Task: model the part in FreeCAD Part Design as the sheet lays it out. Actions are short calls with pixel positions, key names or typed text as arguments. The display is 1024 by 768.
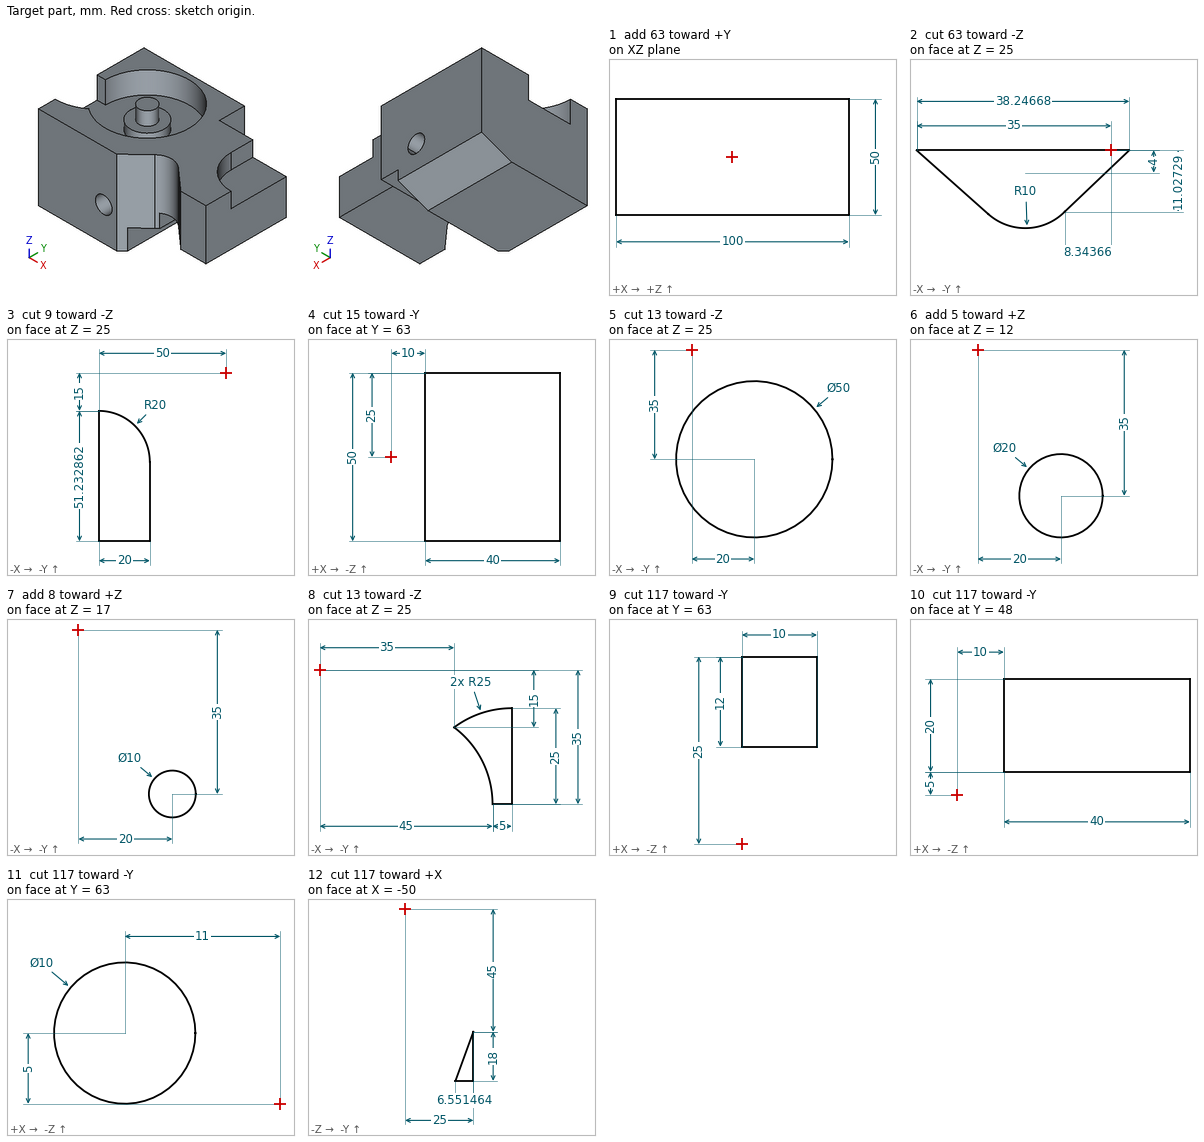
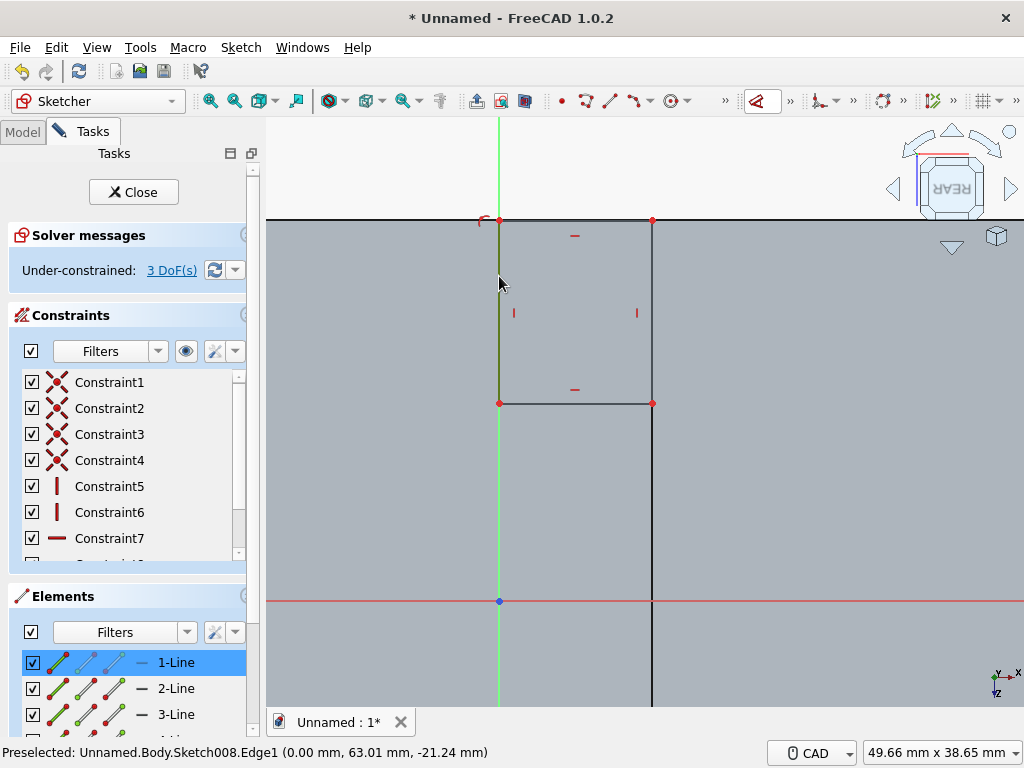
click(776, 102)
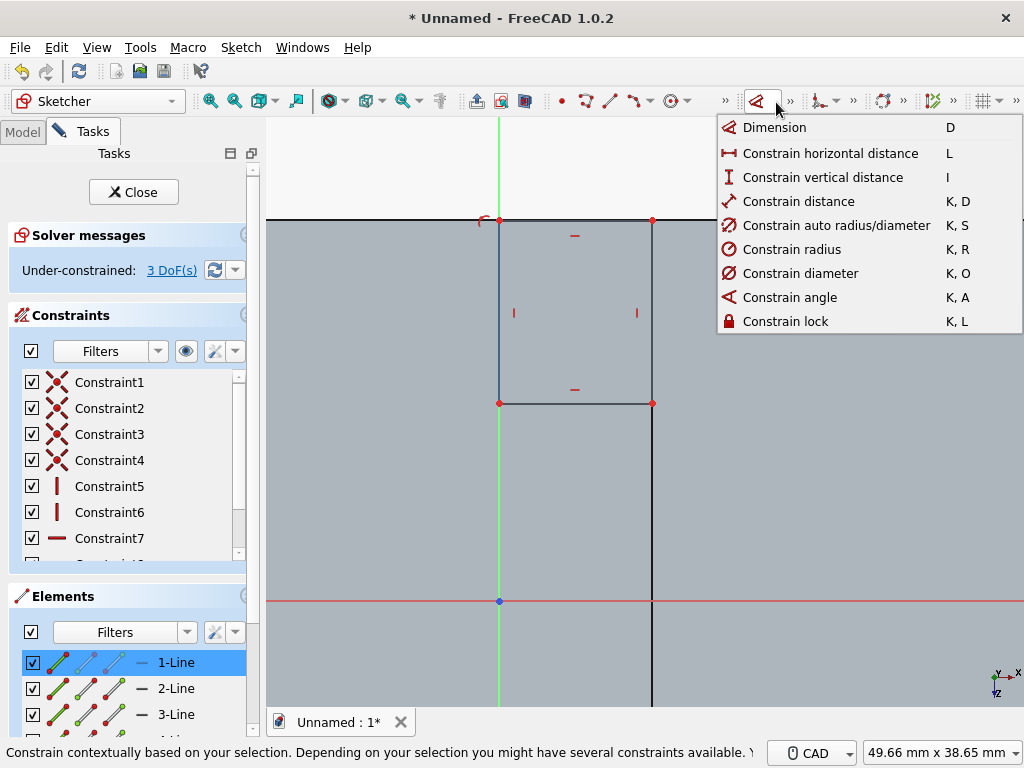
click(870, 177)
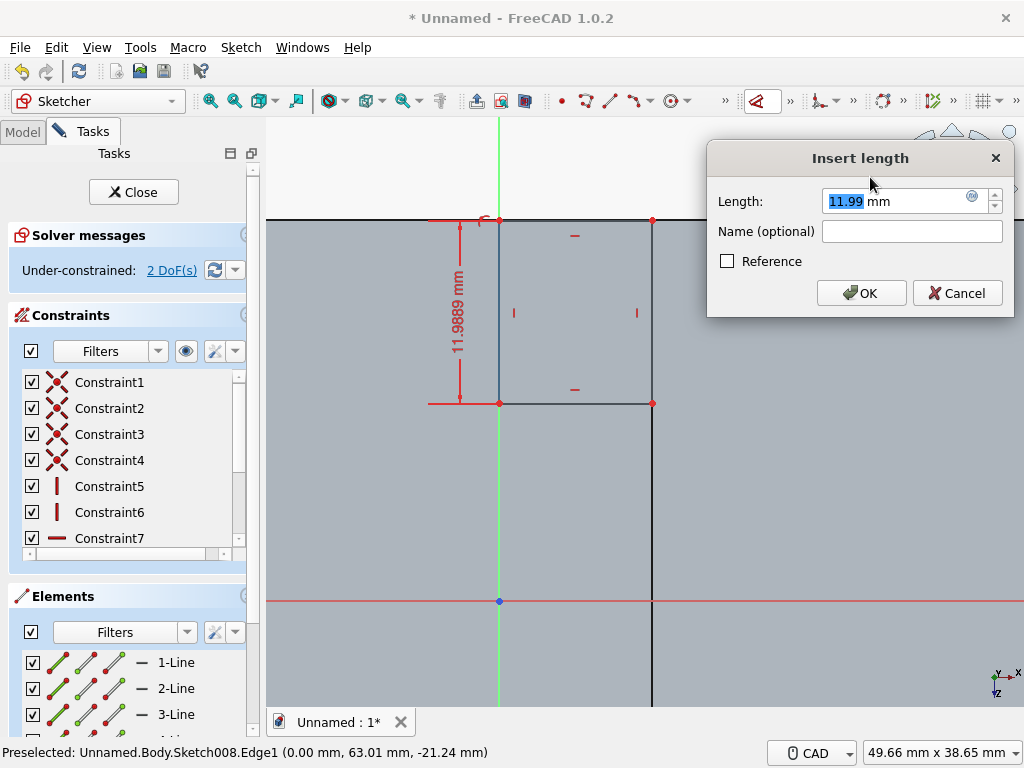
text(12)
key(Return)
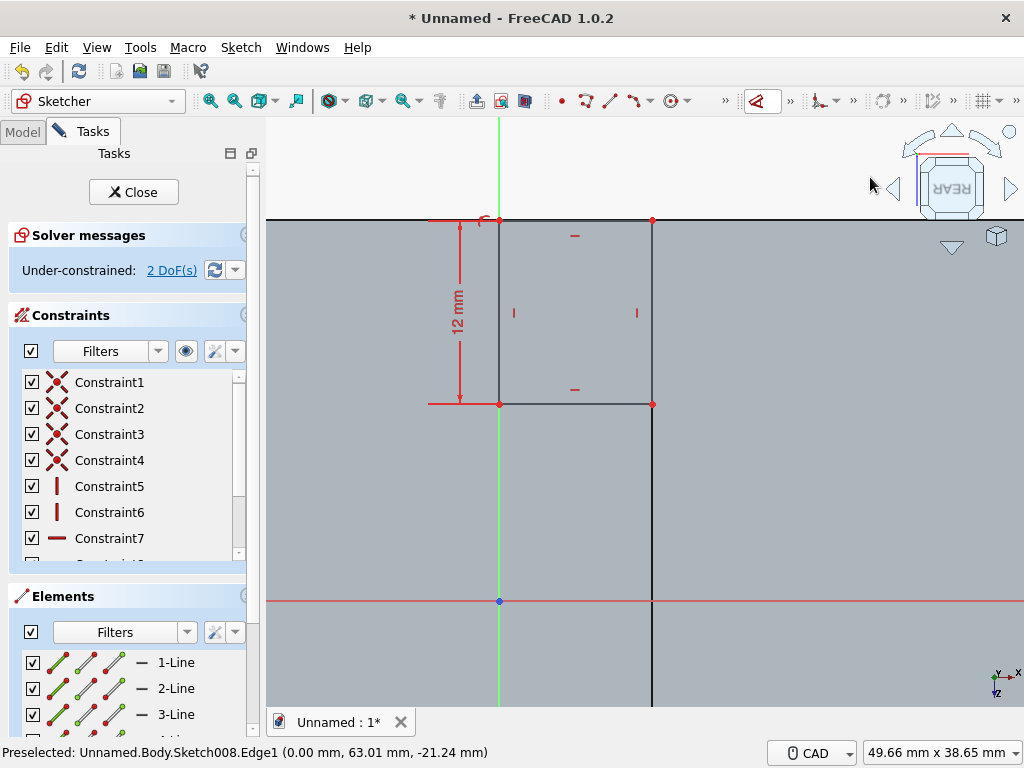
click(545, 404)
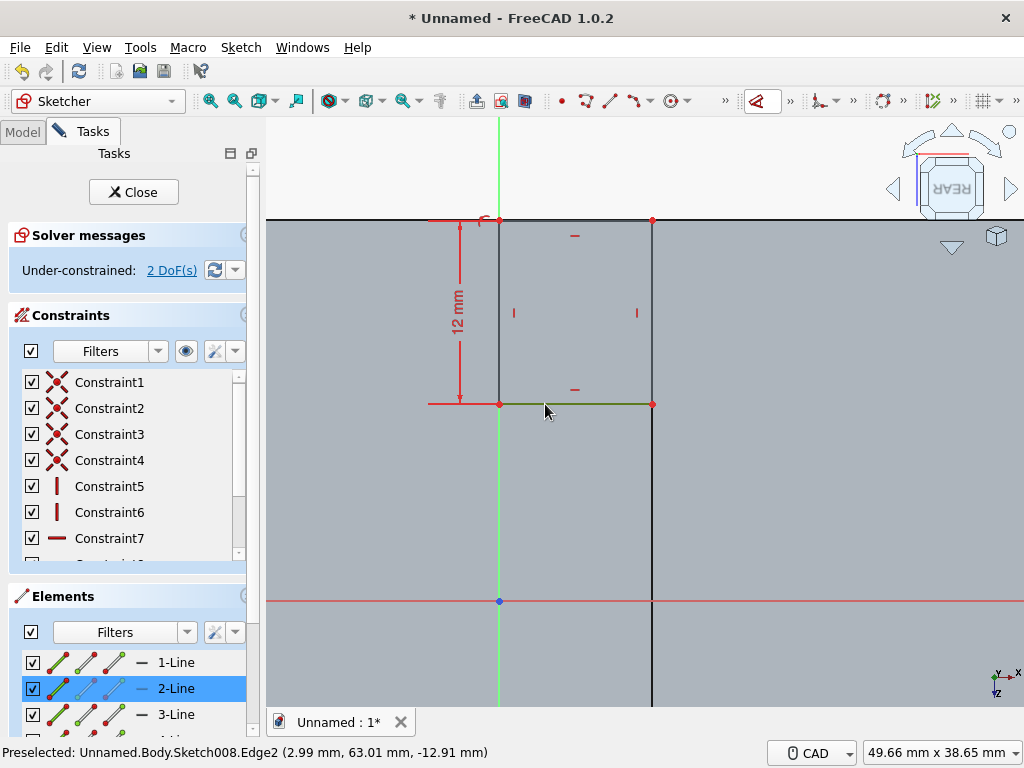
key(l)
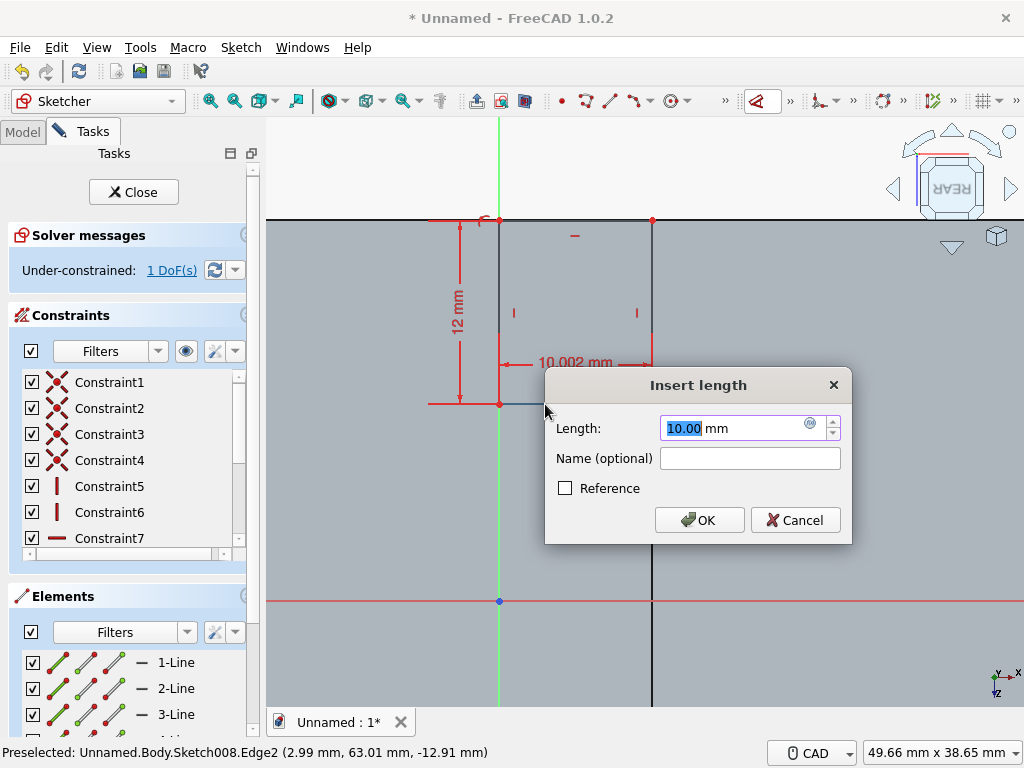
text(10)
key(Return)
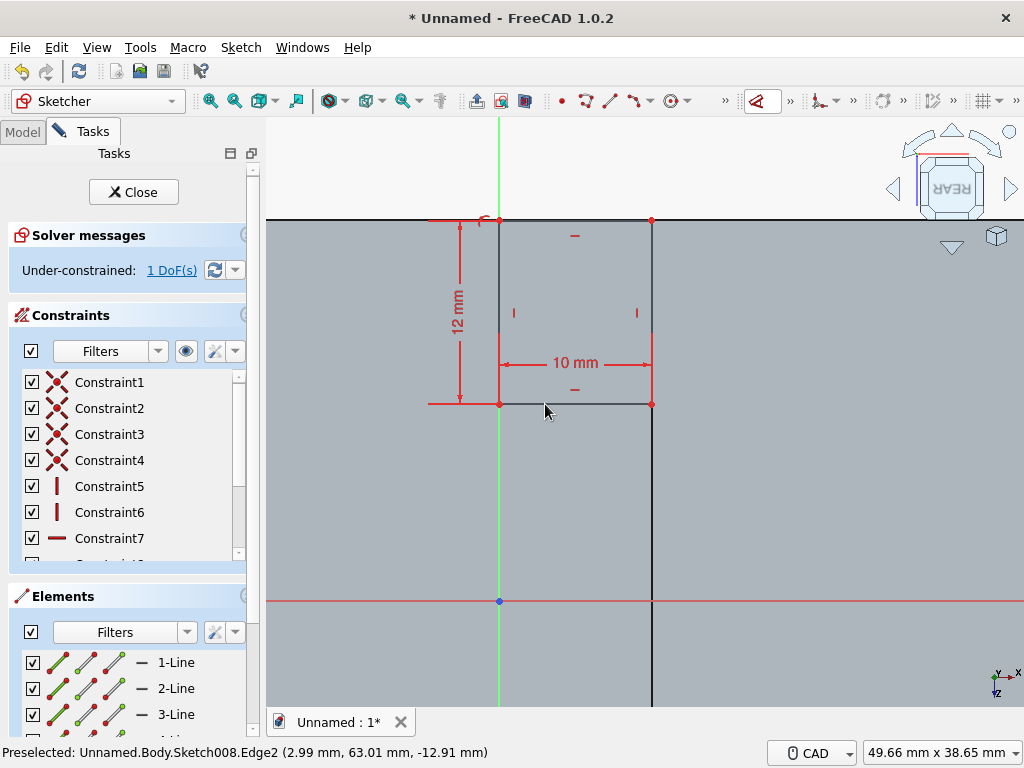
click(499, 221)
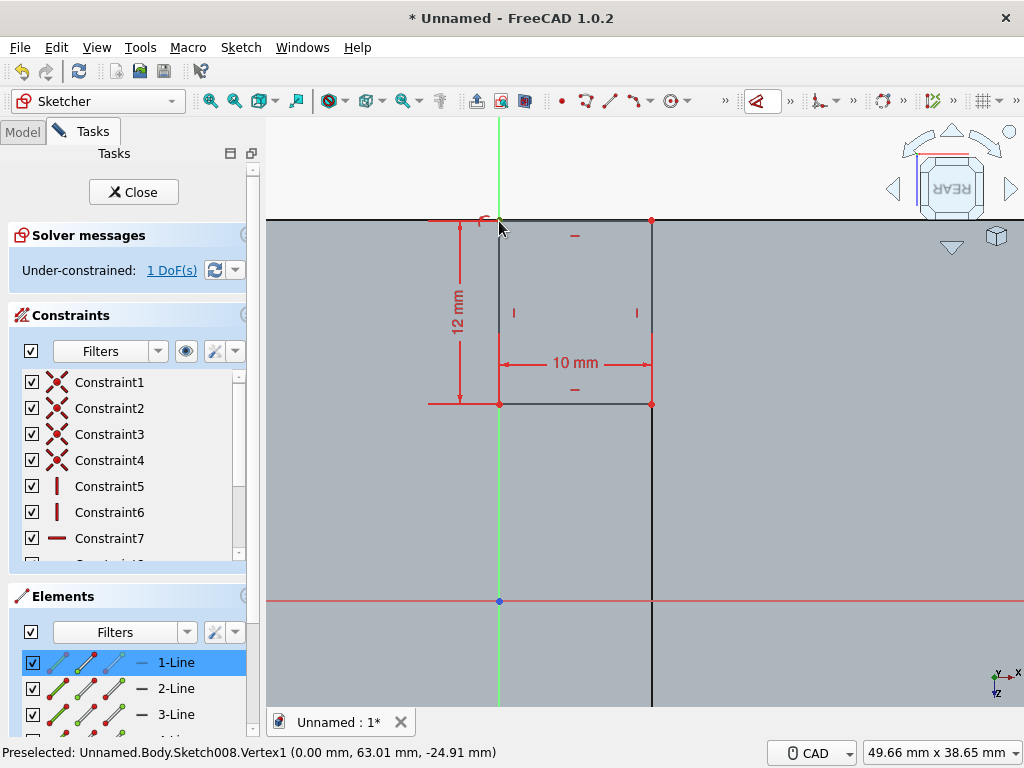
click(776, 102)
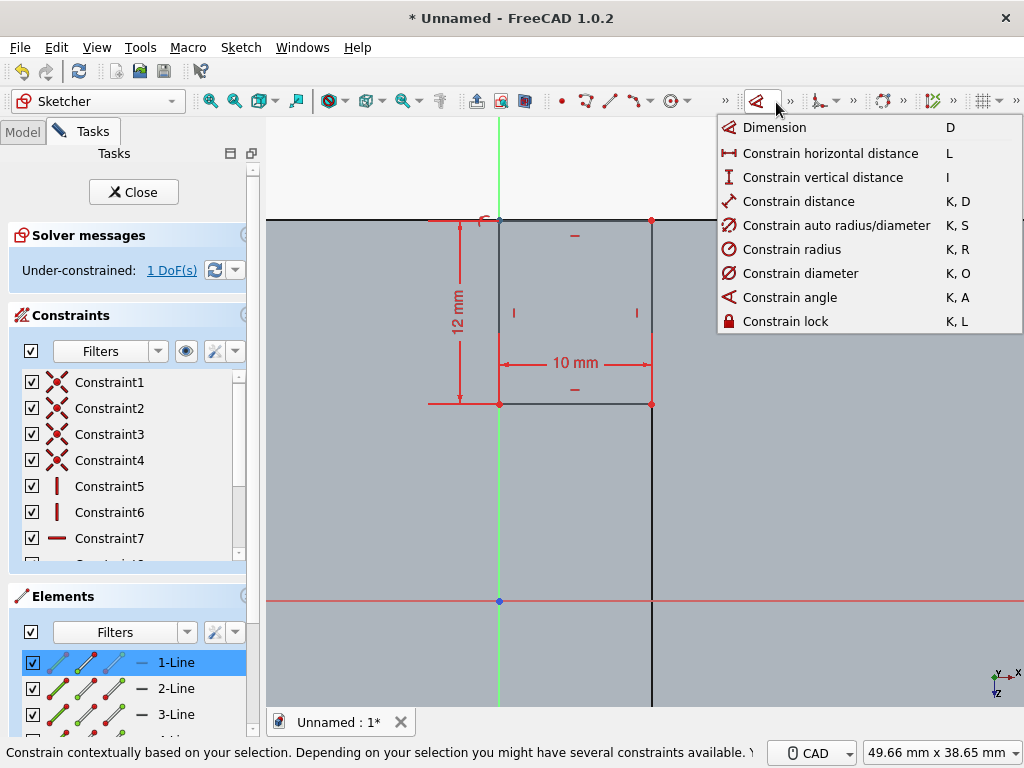
click(870, 177)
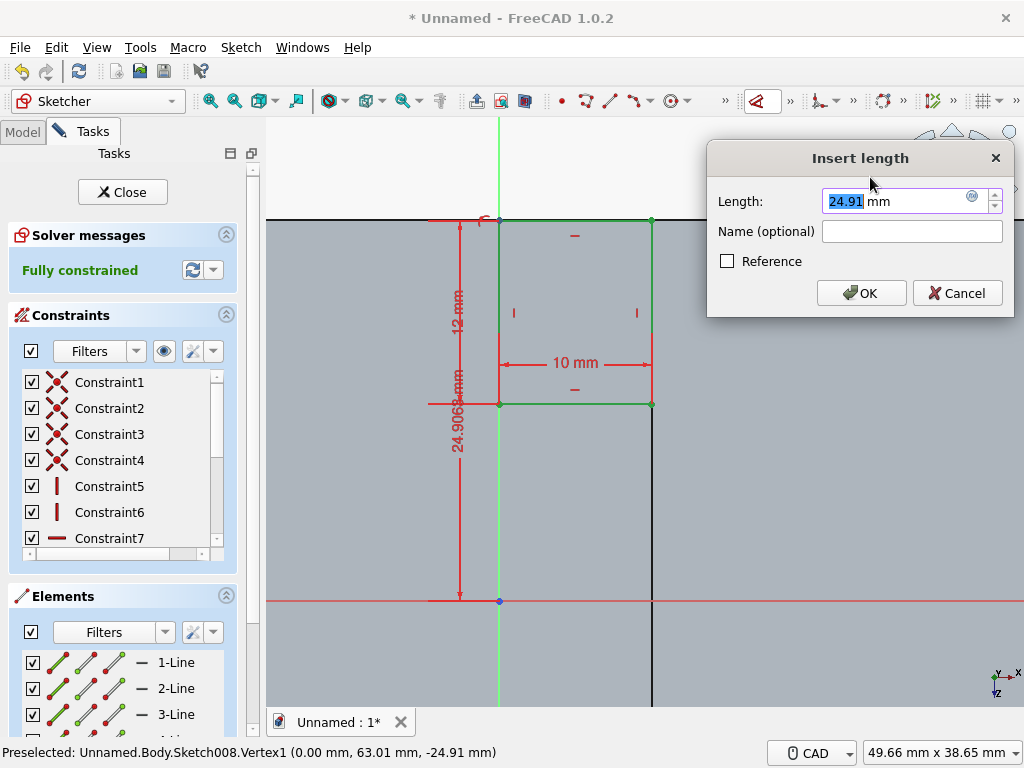
text(25)
key(Return)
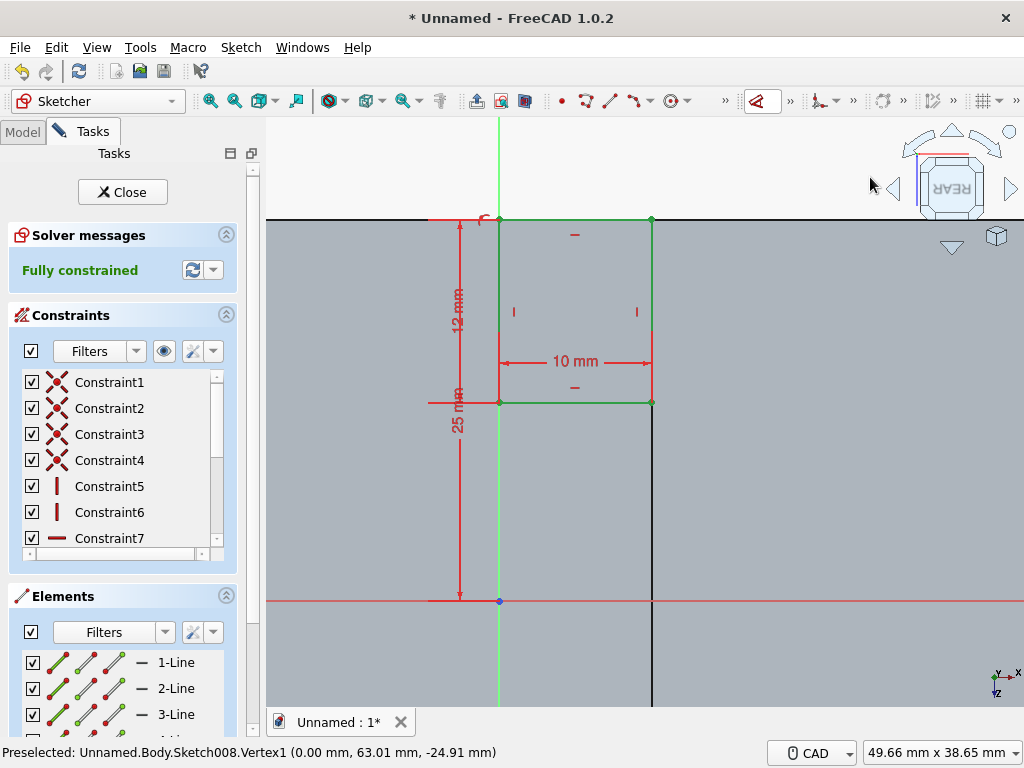
click(123, 192)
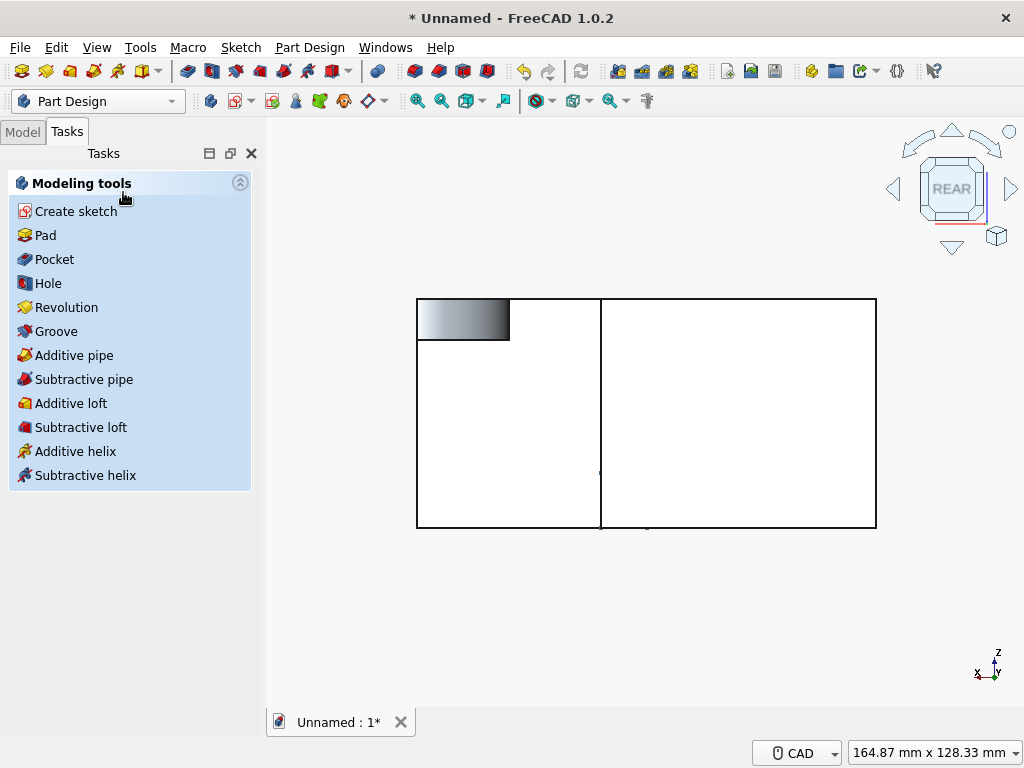
click(188, 72)